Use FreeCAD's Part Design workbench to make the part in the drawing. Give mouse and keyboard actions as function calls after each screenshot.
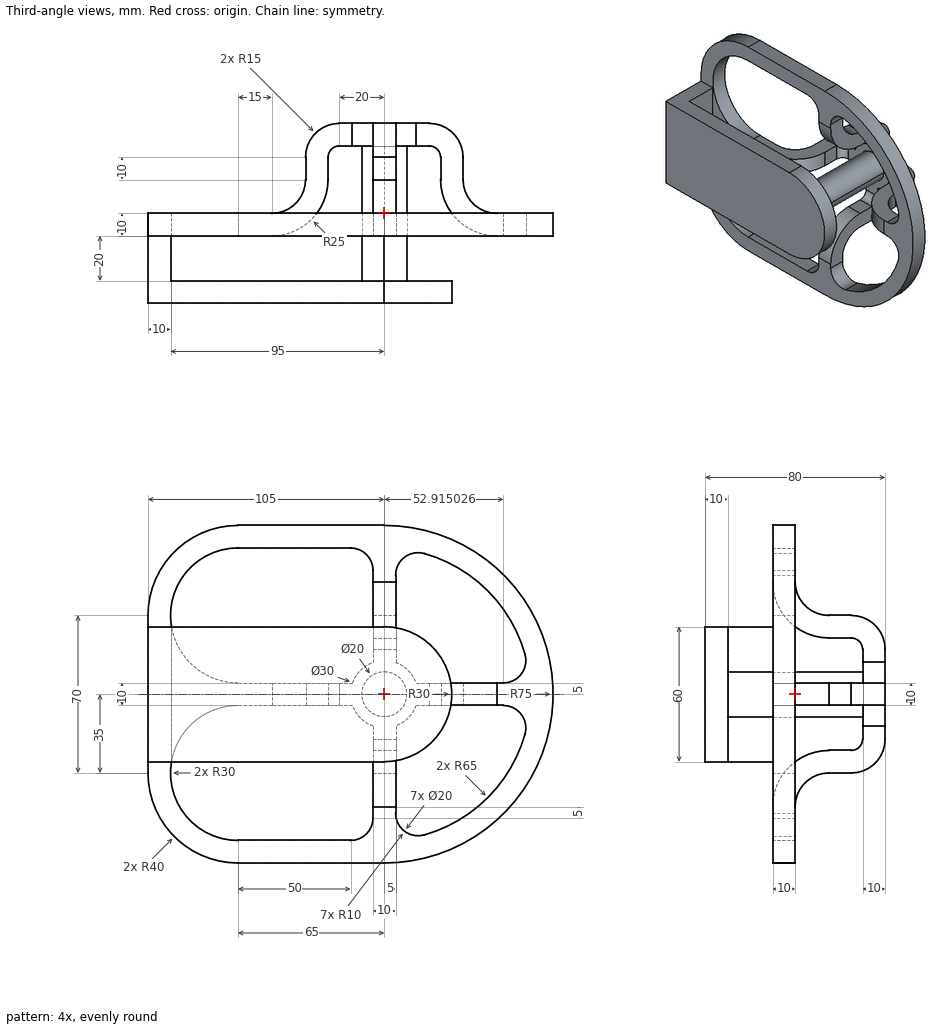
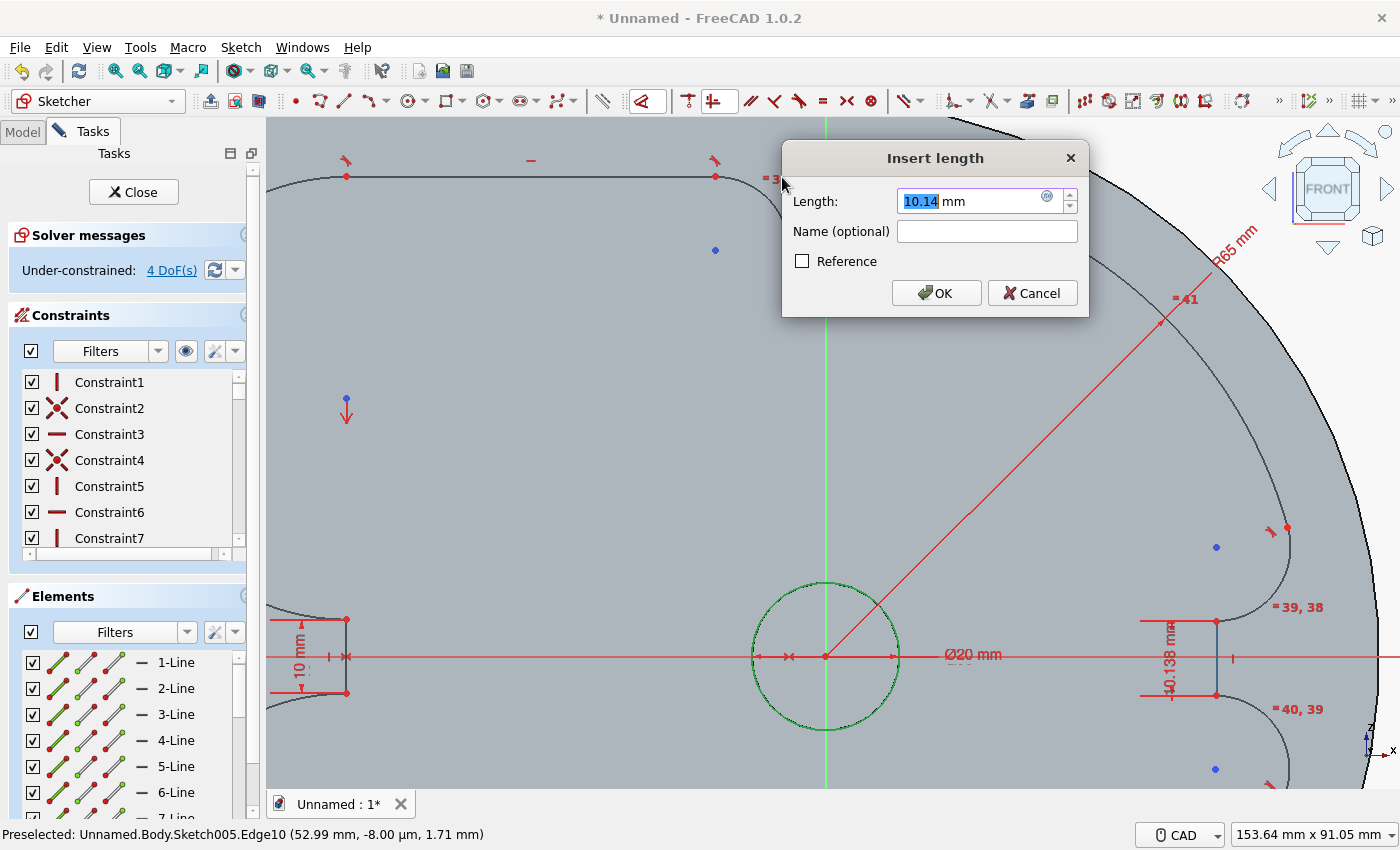
text(10)
key(Return)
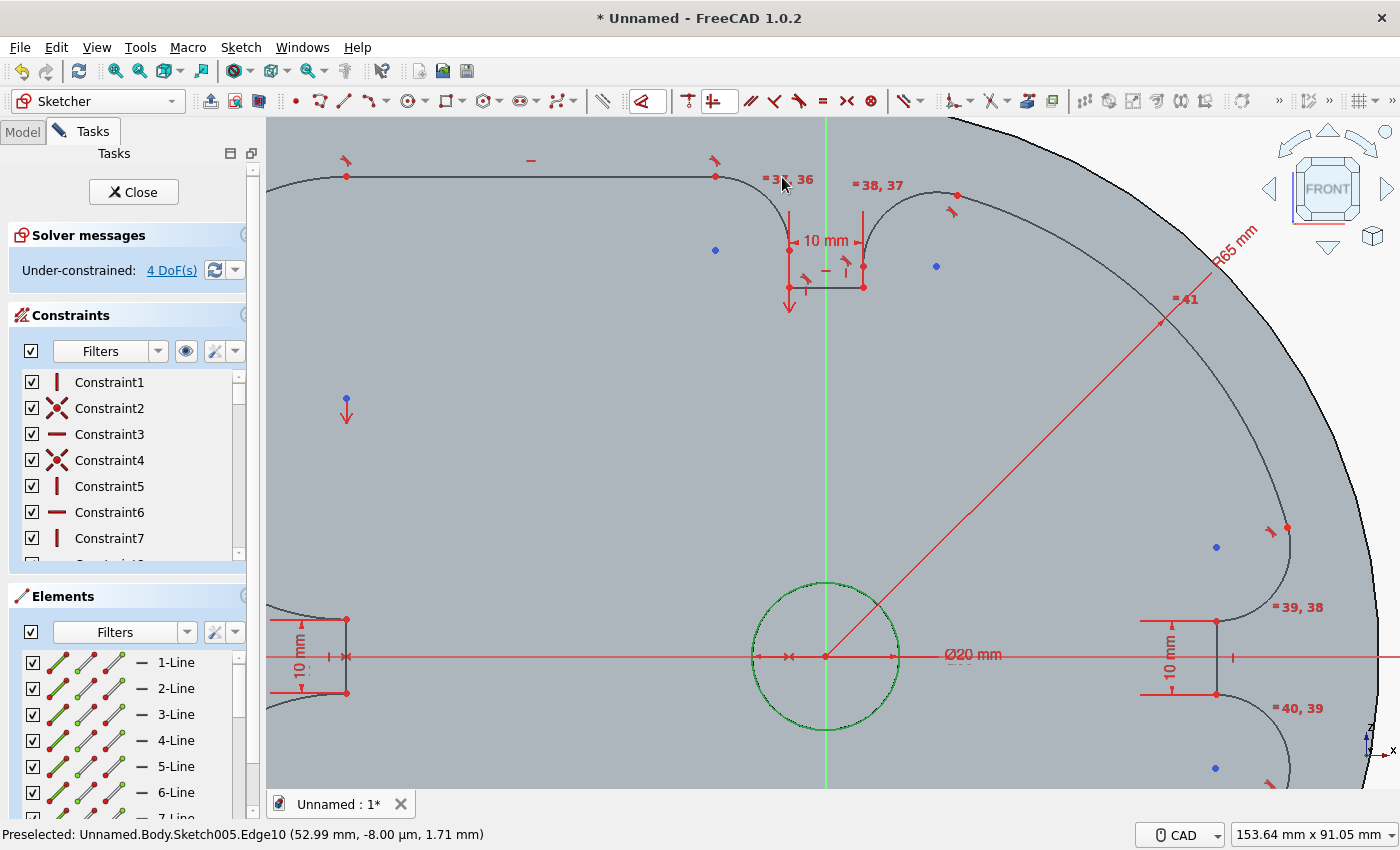
scroll(812, 287, down, 4)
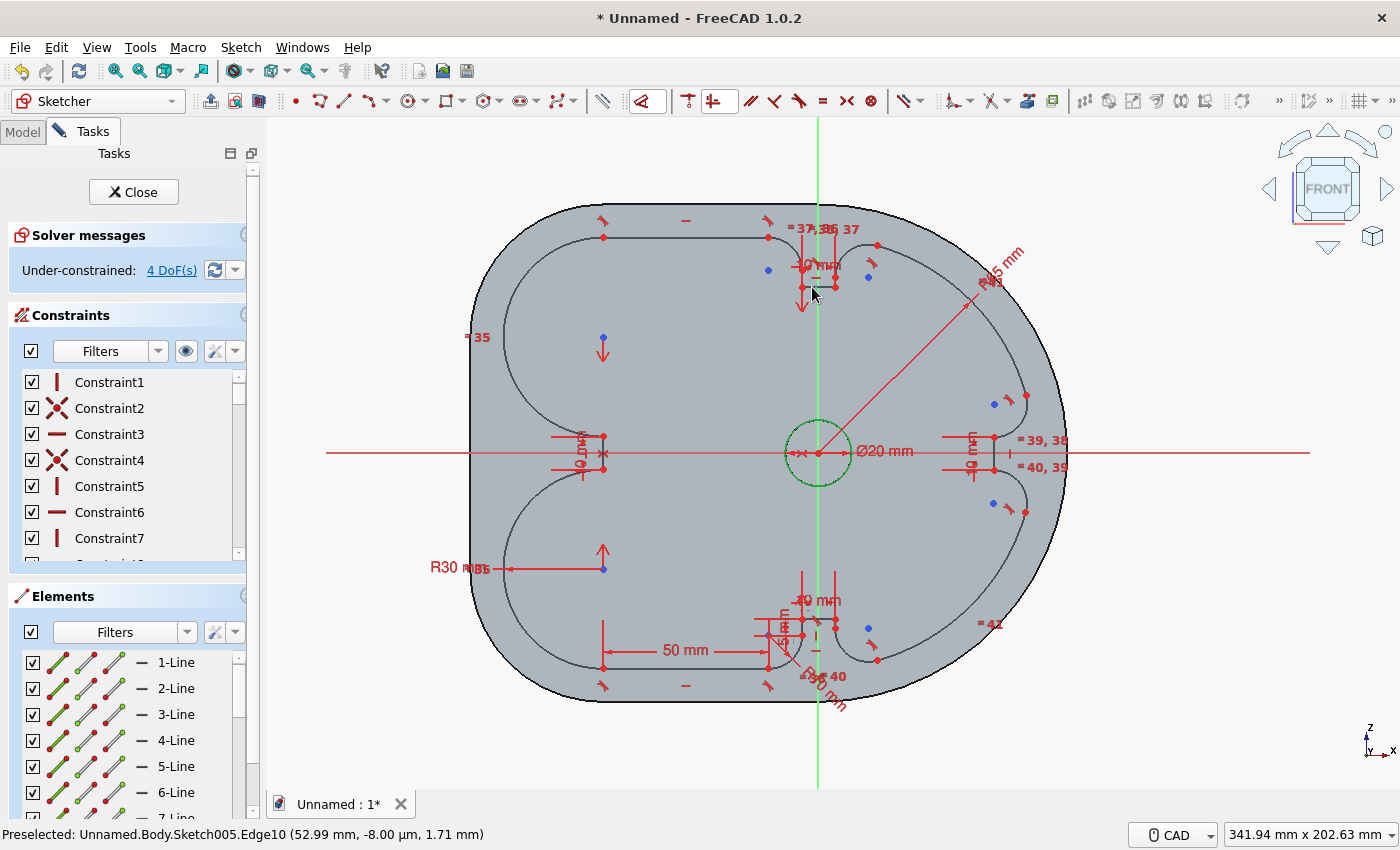
scroll(835, 629, up, 5)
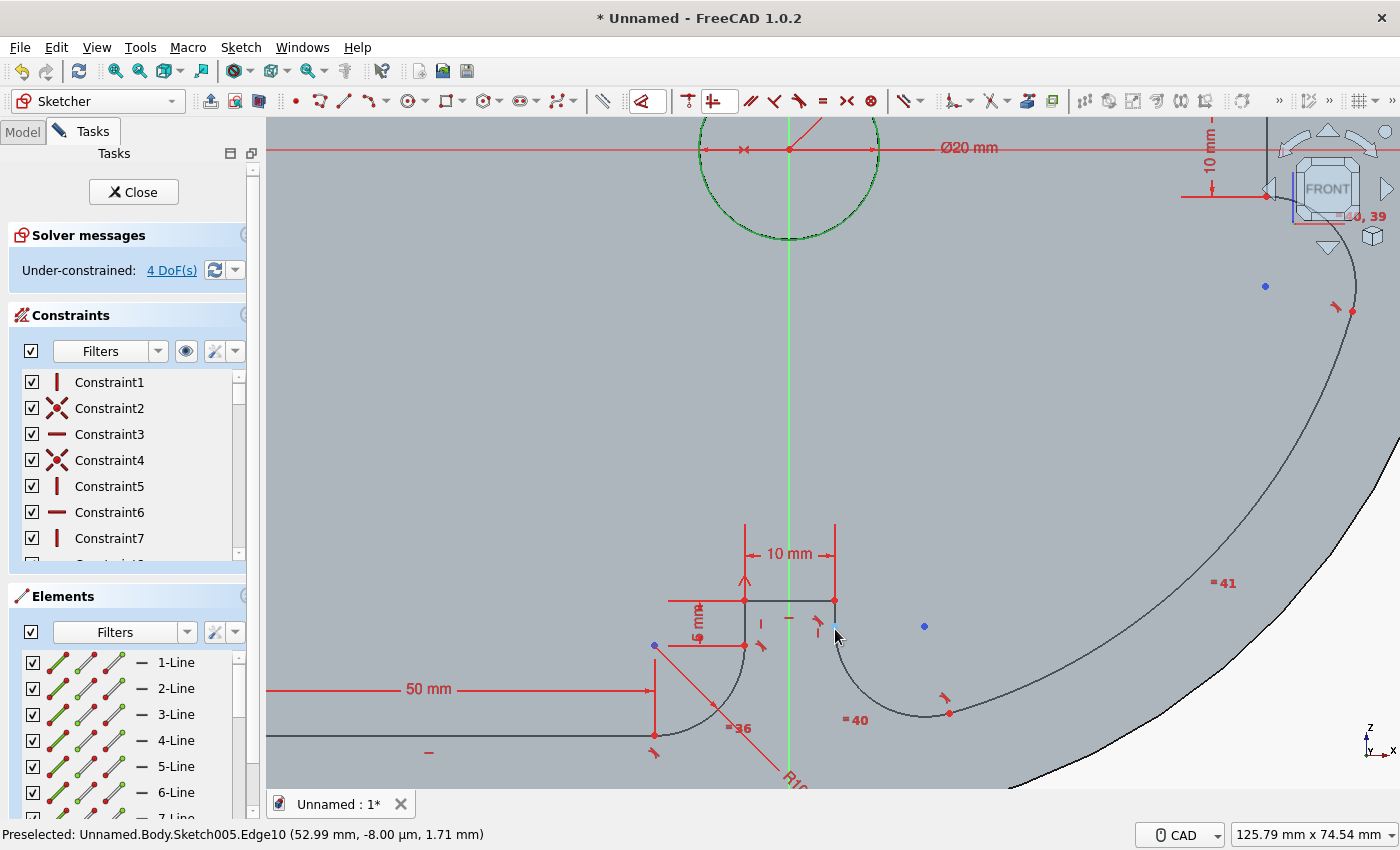
click(835, 627)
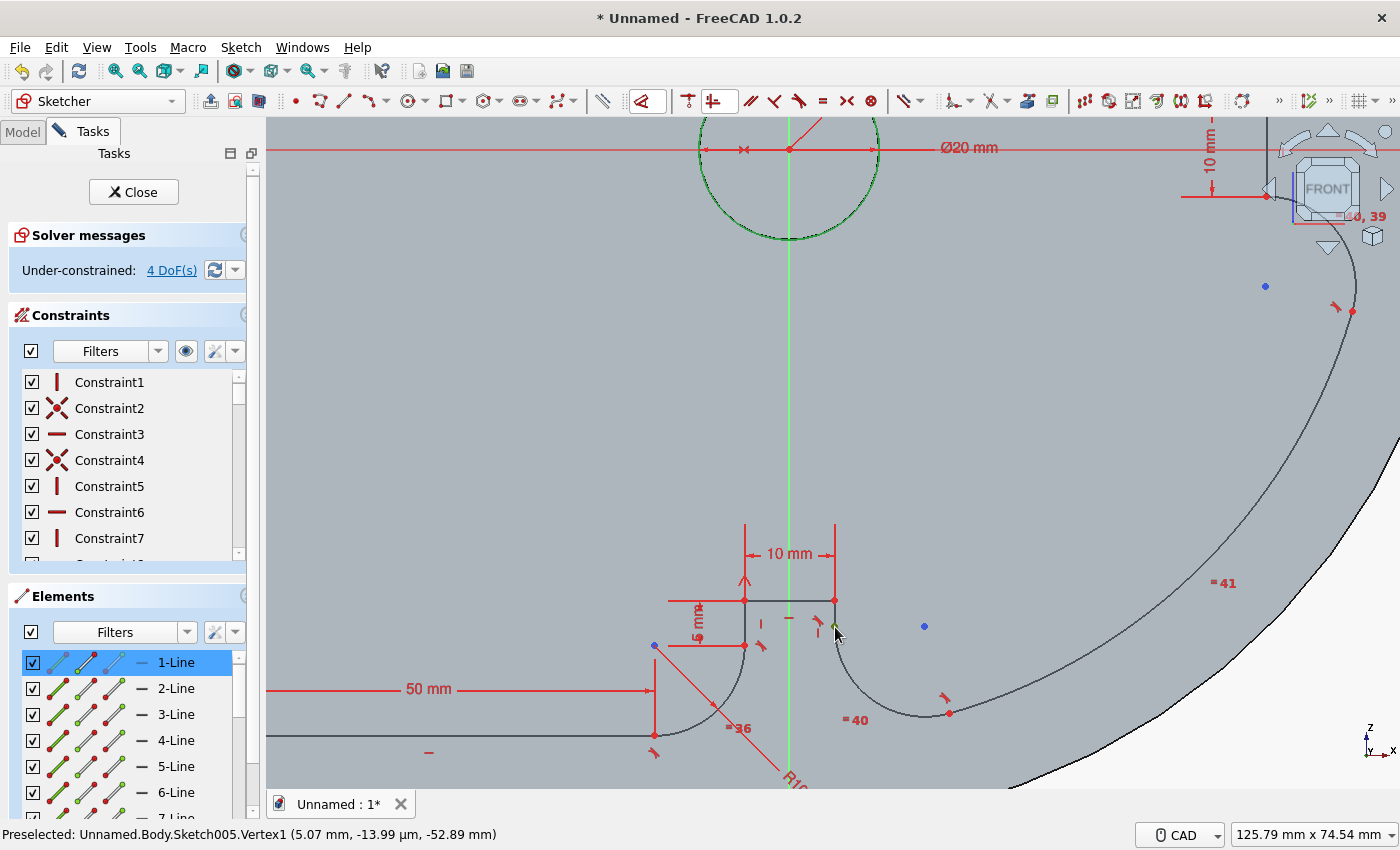
click(660, 102)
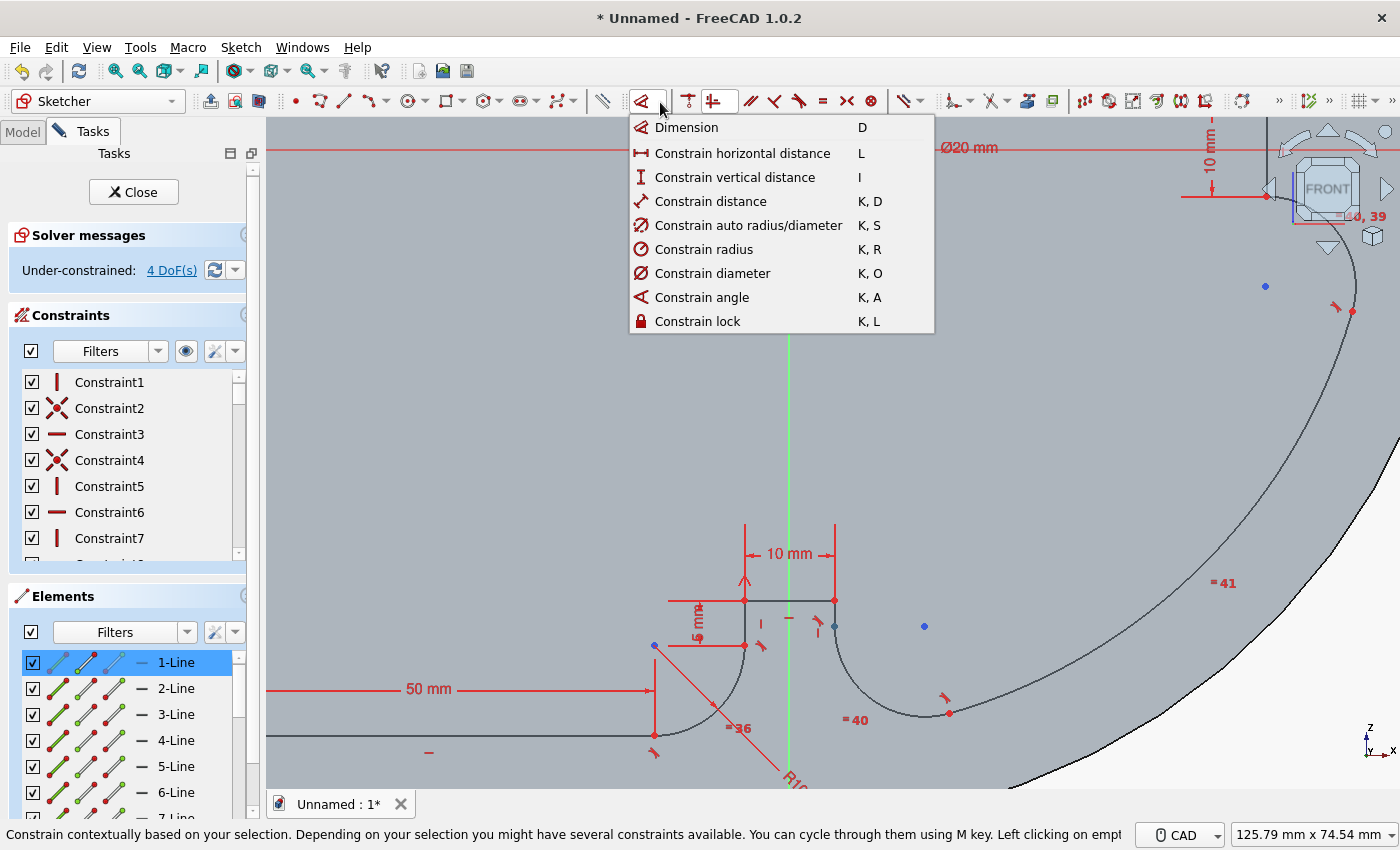
click(782, 153)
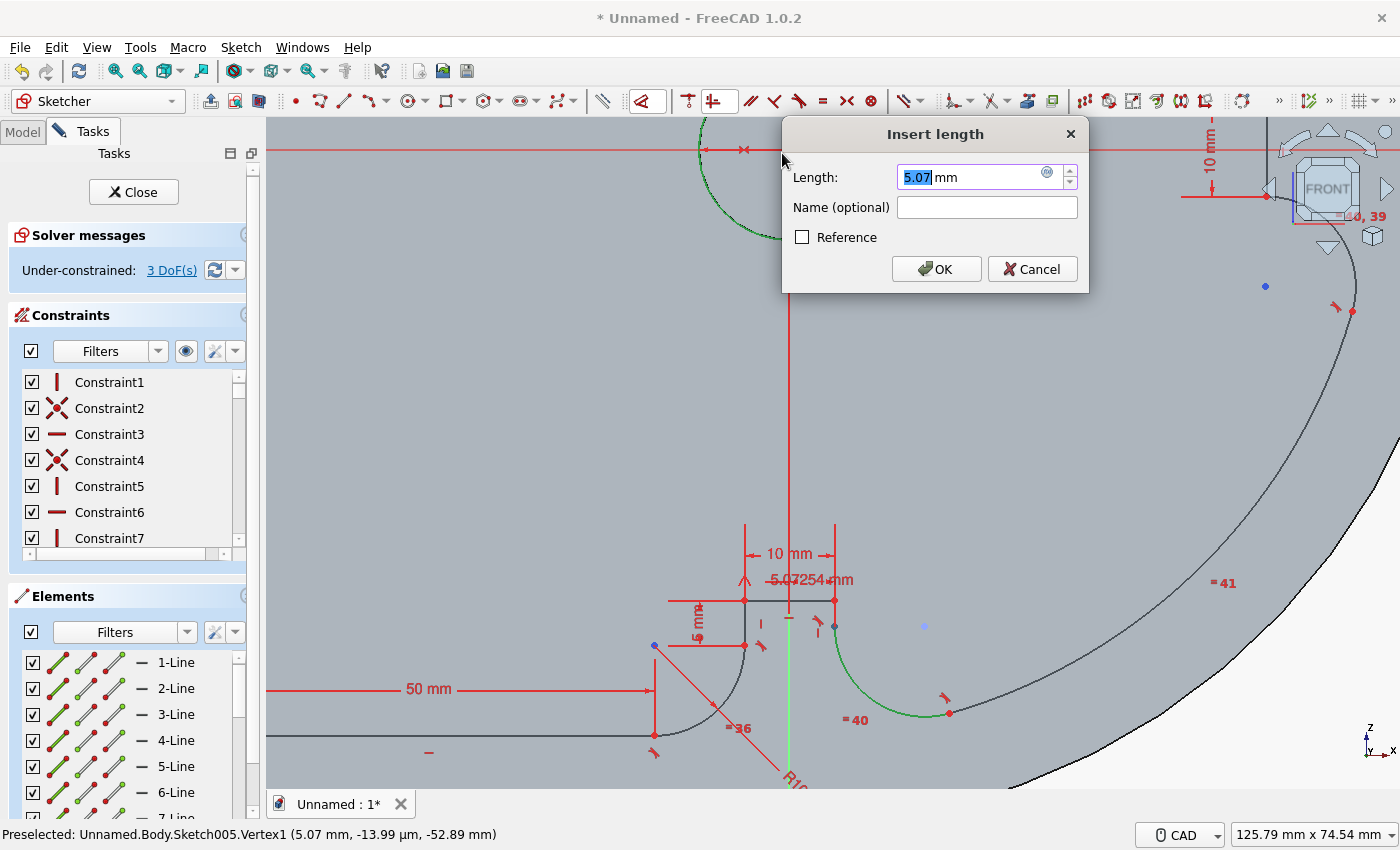
text(5)
key(Return)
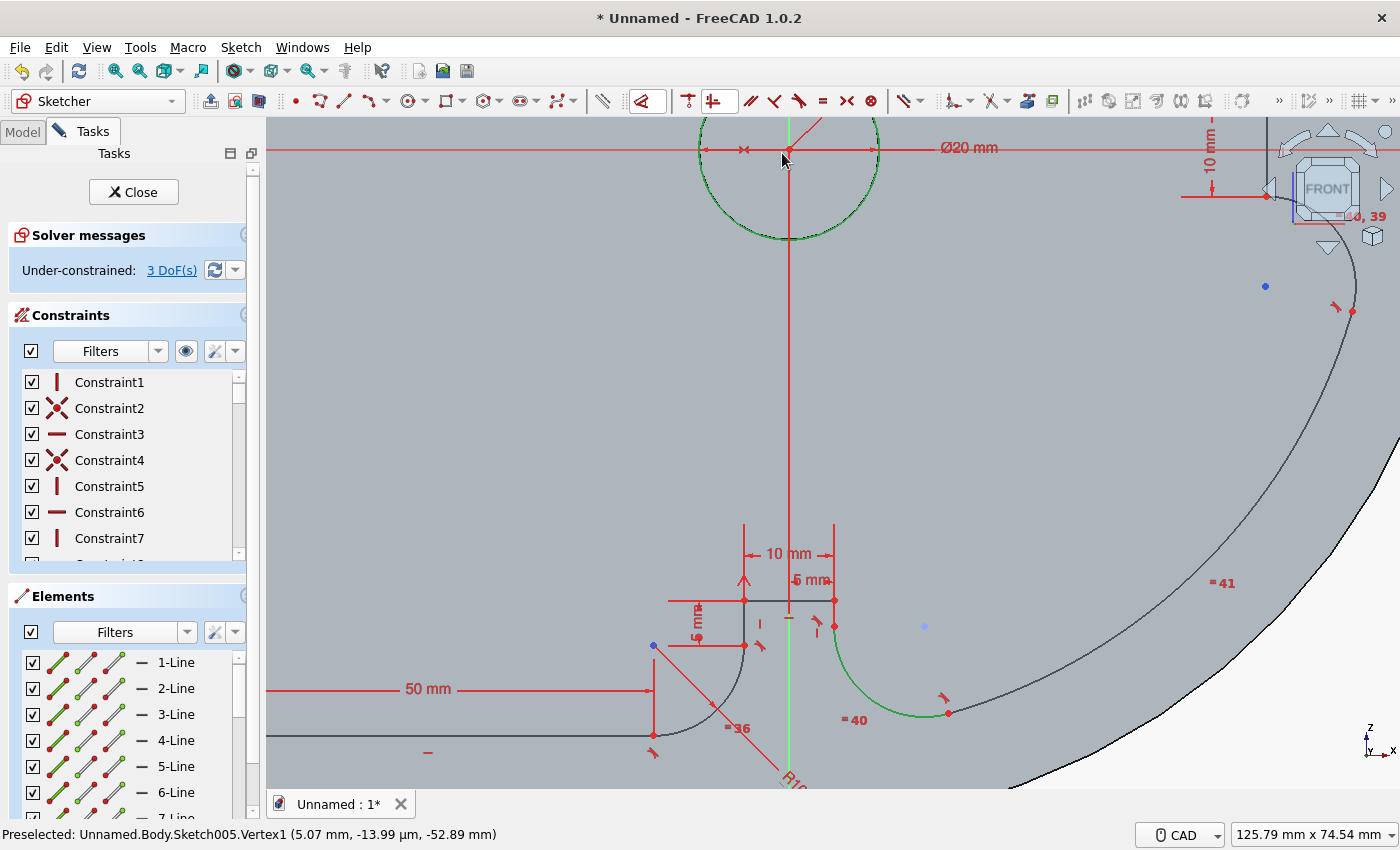
scroll(835, 629, down, 5)